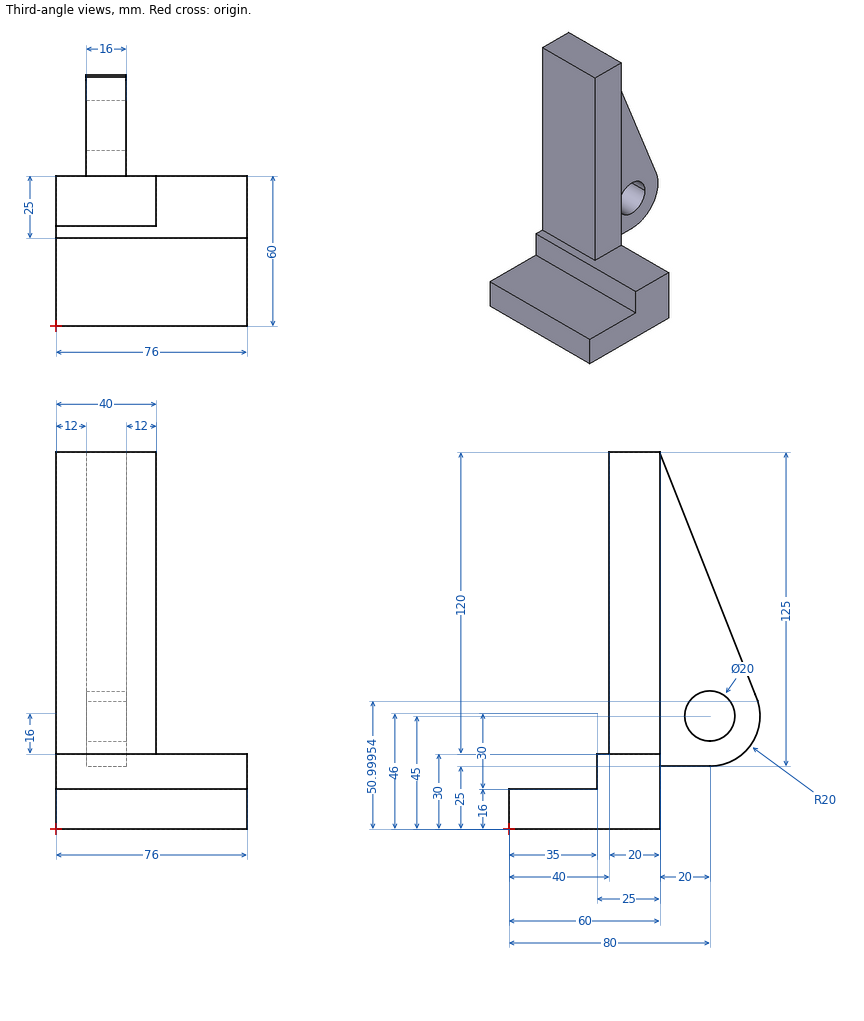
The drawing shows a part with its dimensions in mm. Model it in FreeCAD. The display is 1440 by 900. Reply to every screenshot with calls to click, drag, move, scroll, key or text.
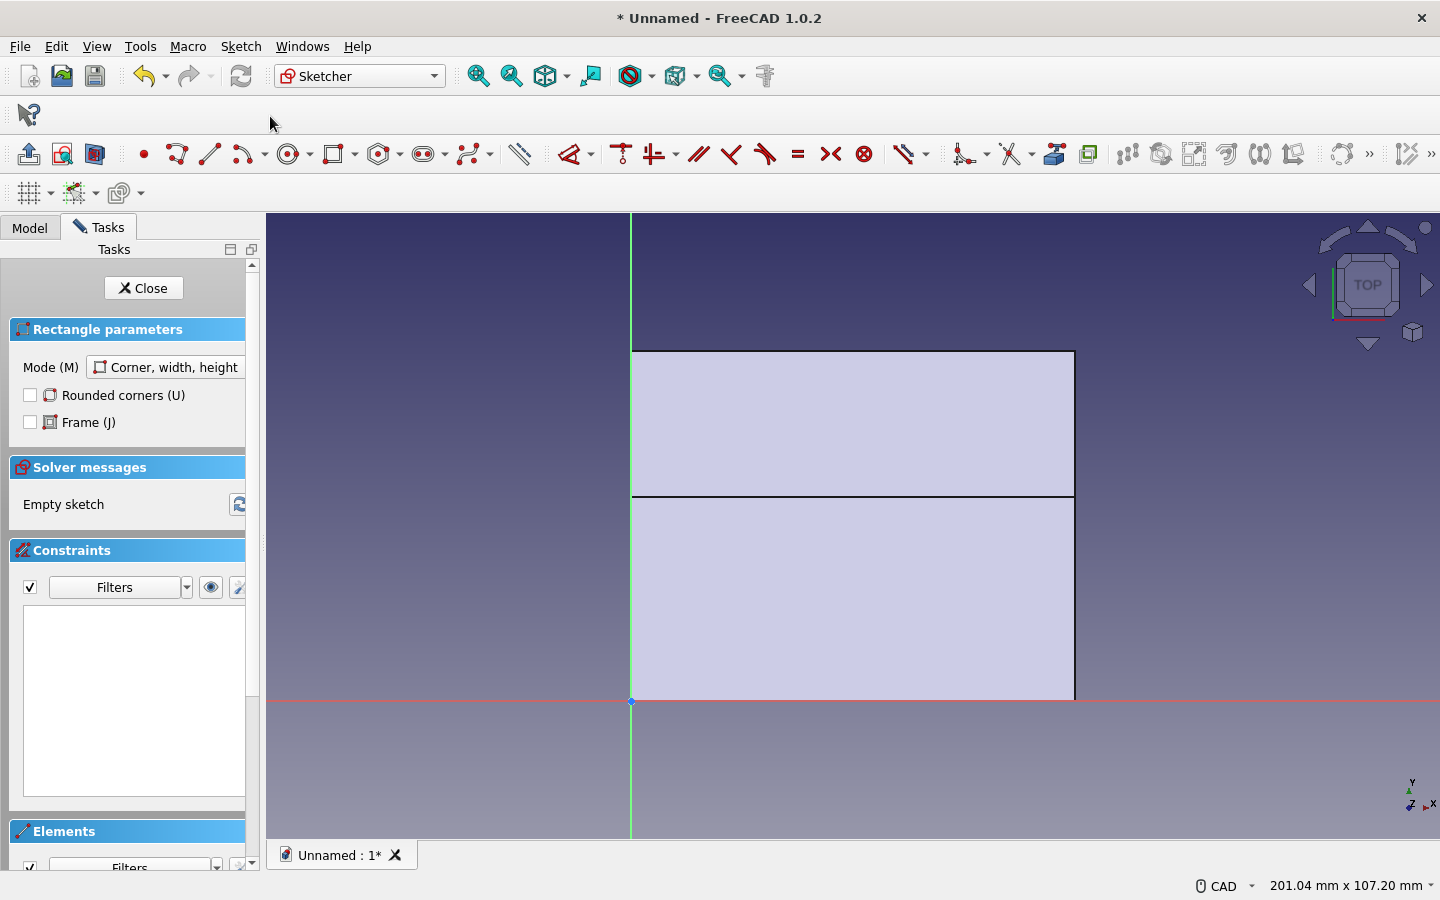
click(631, 351)
click(1075, 497)
key(Escape)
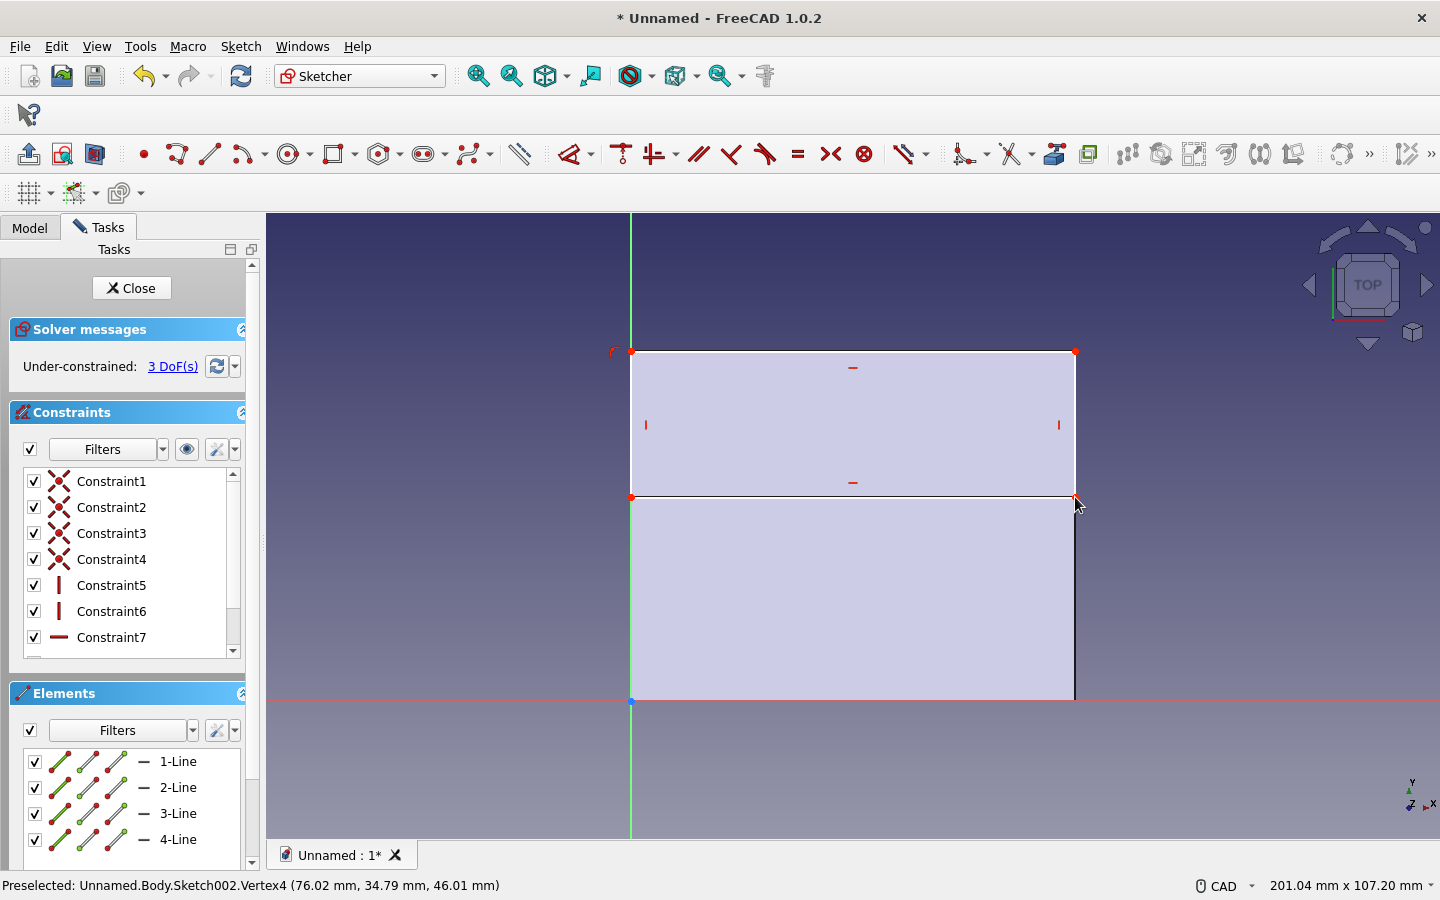
key(d)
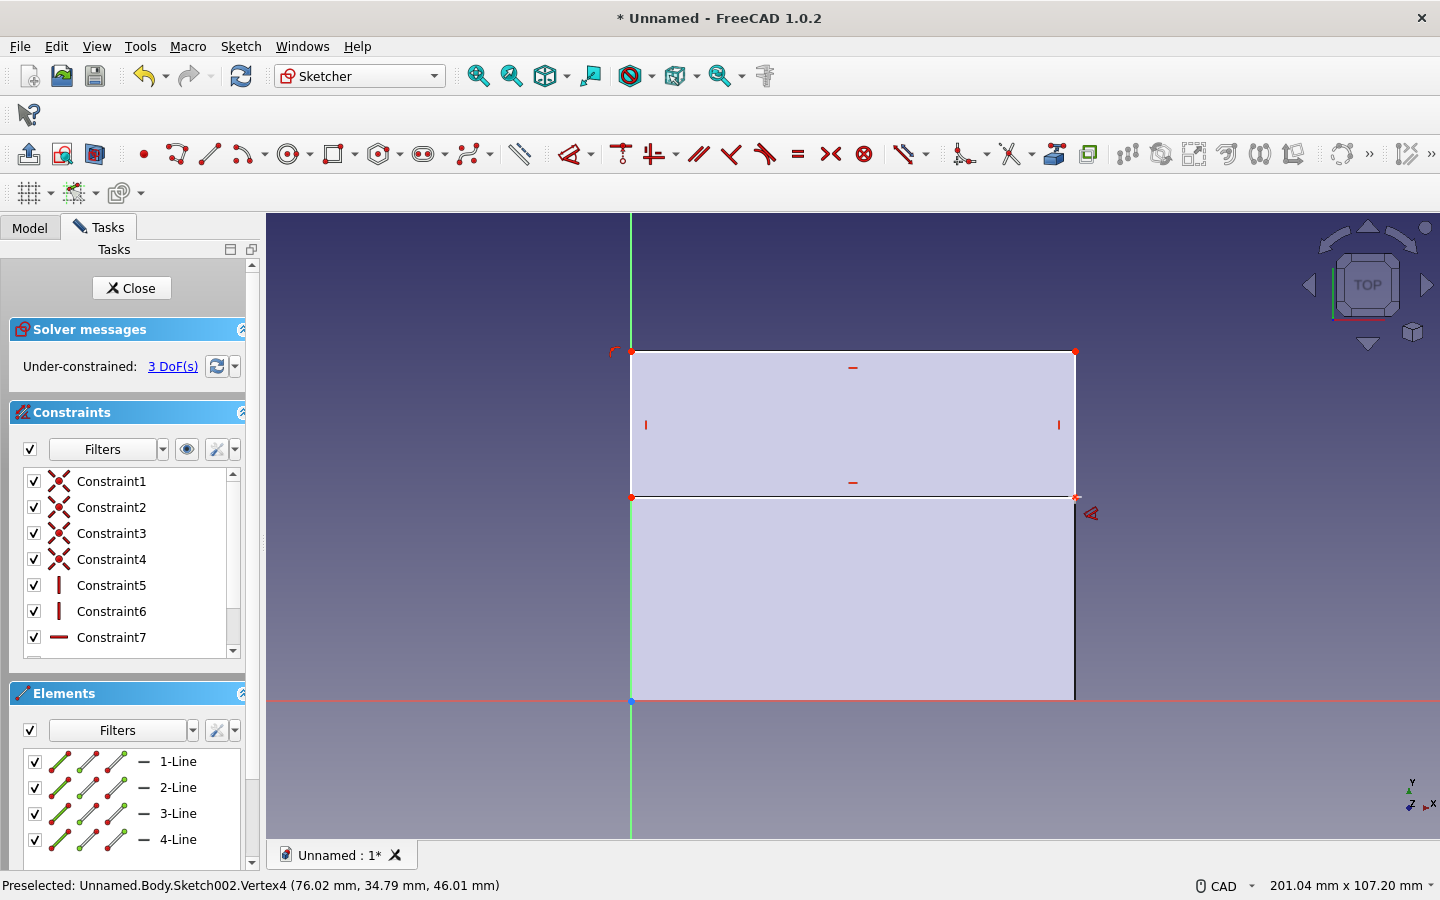
click(631, 396)
click(597, 425)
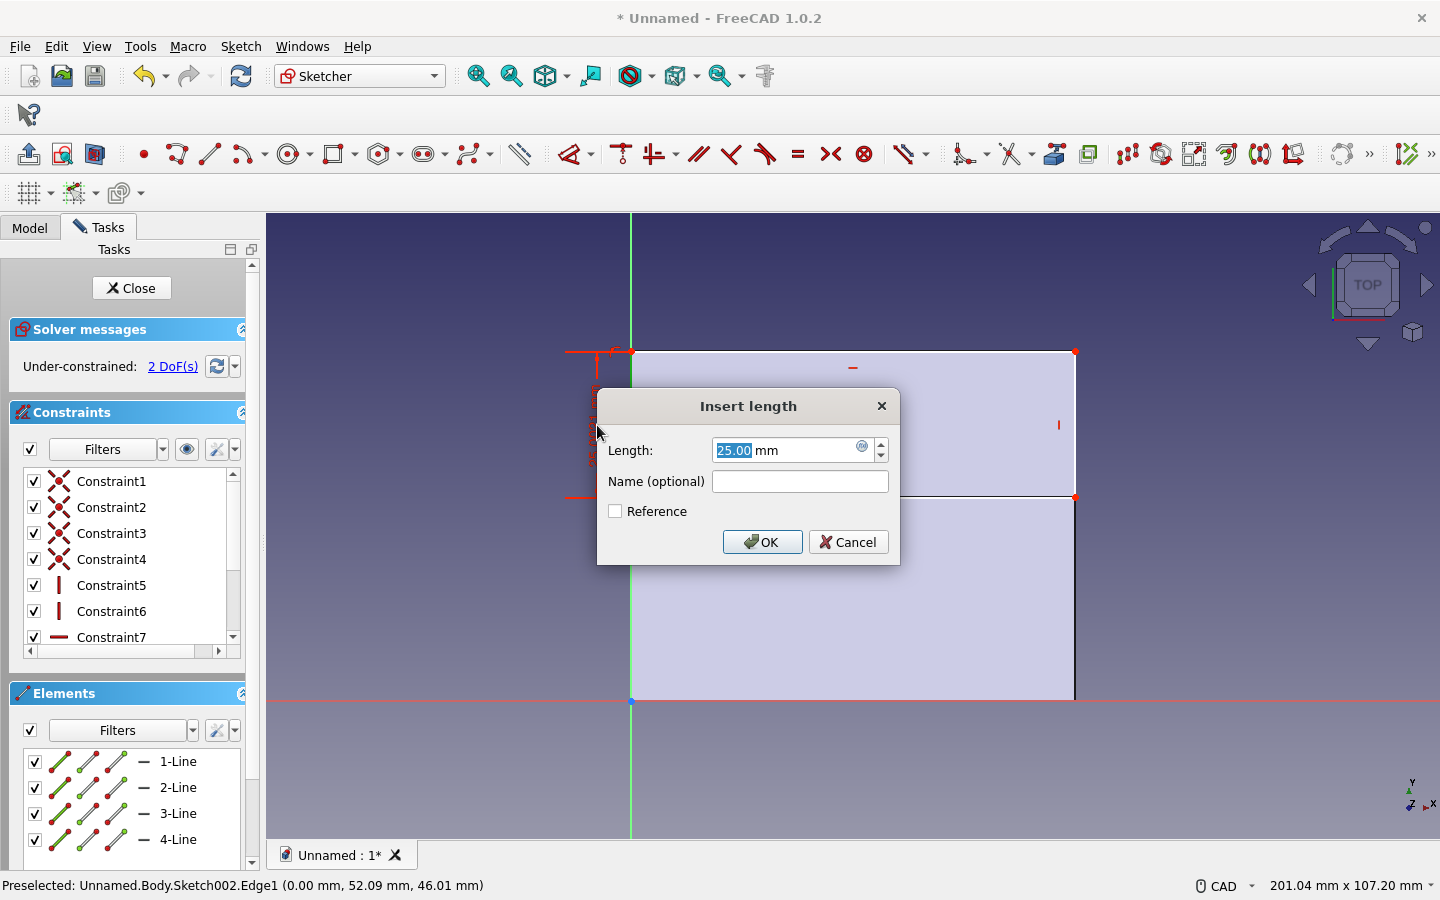
text(25)
key(Return)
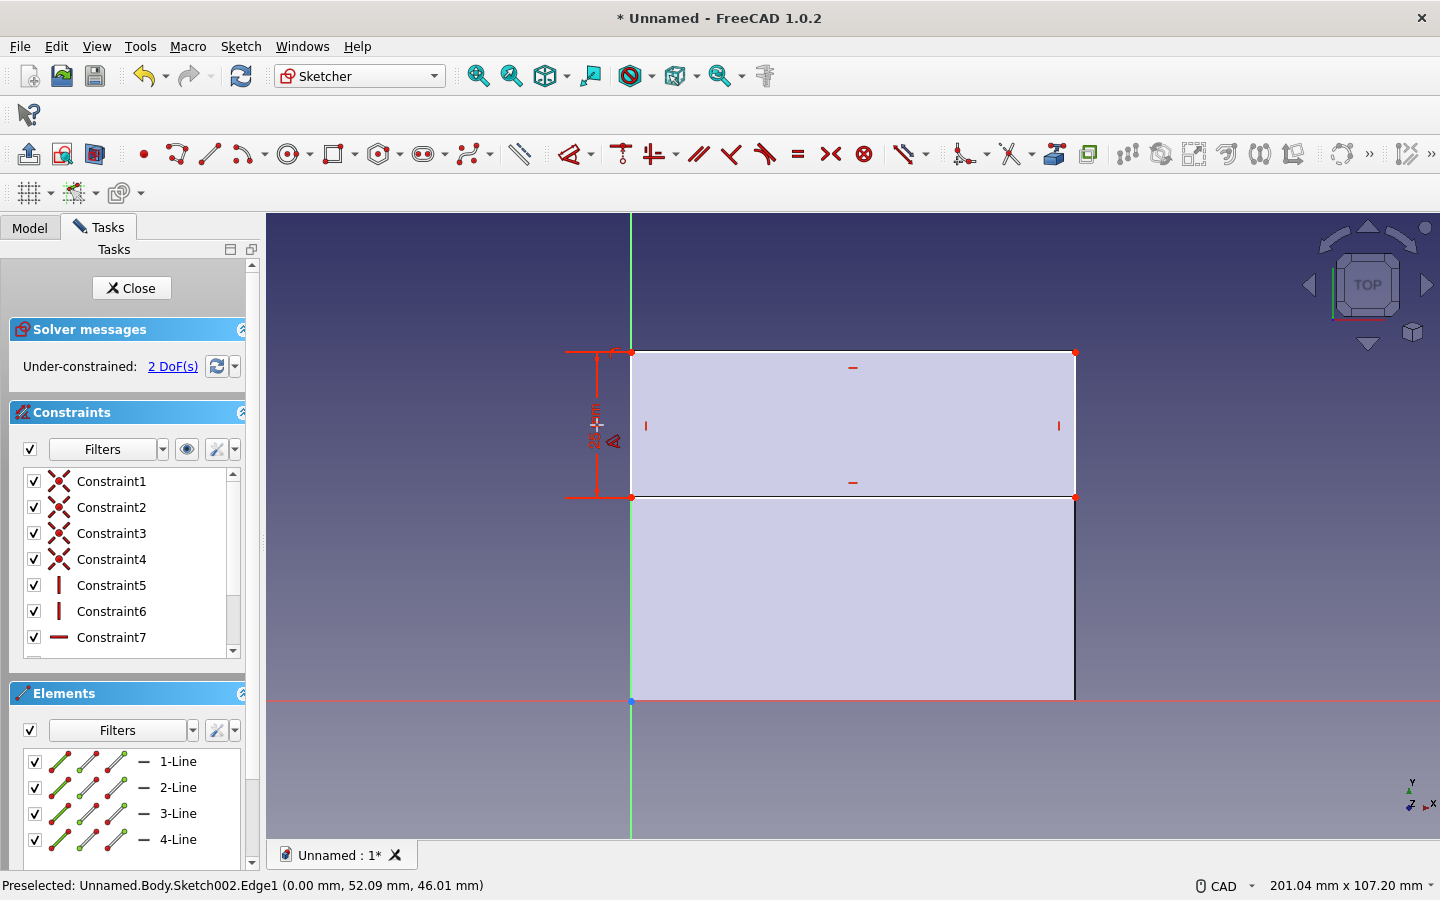
click(764, 498)
click(853, 464)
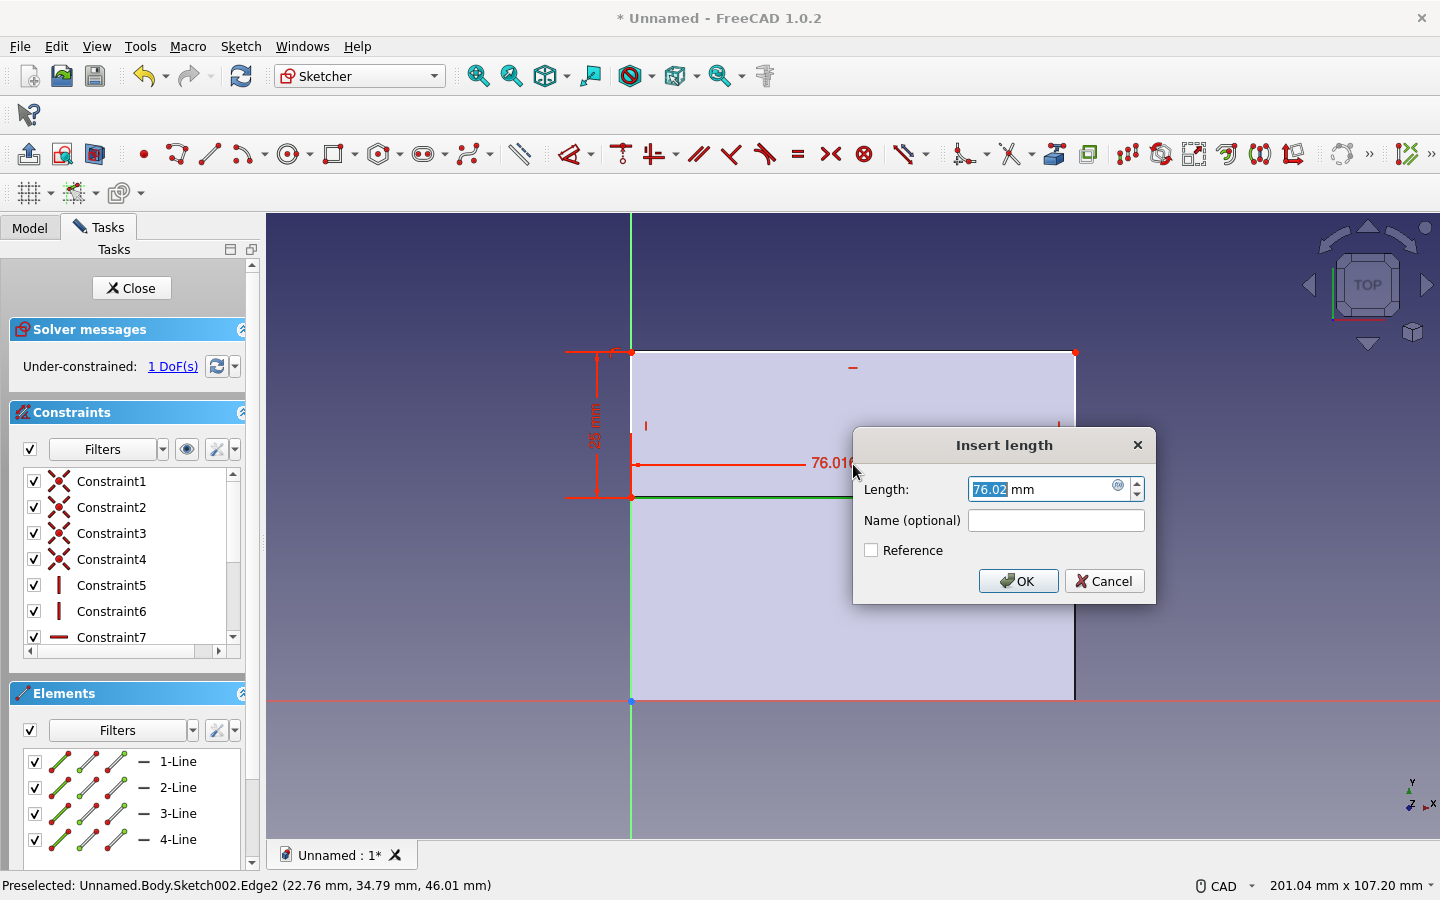
text(76)
key(Return)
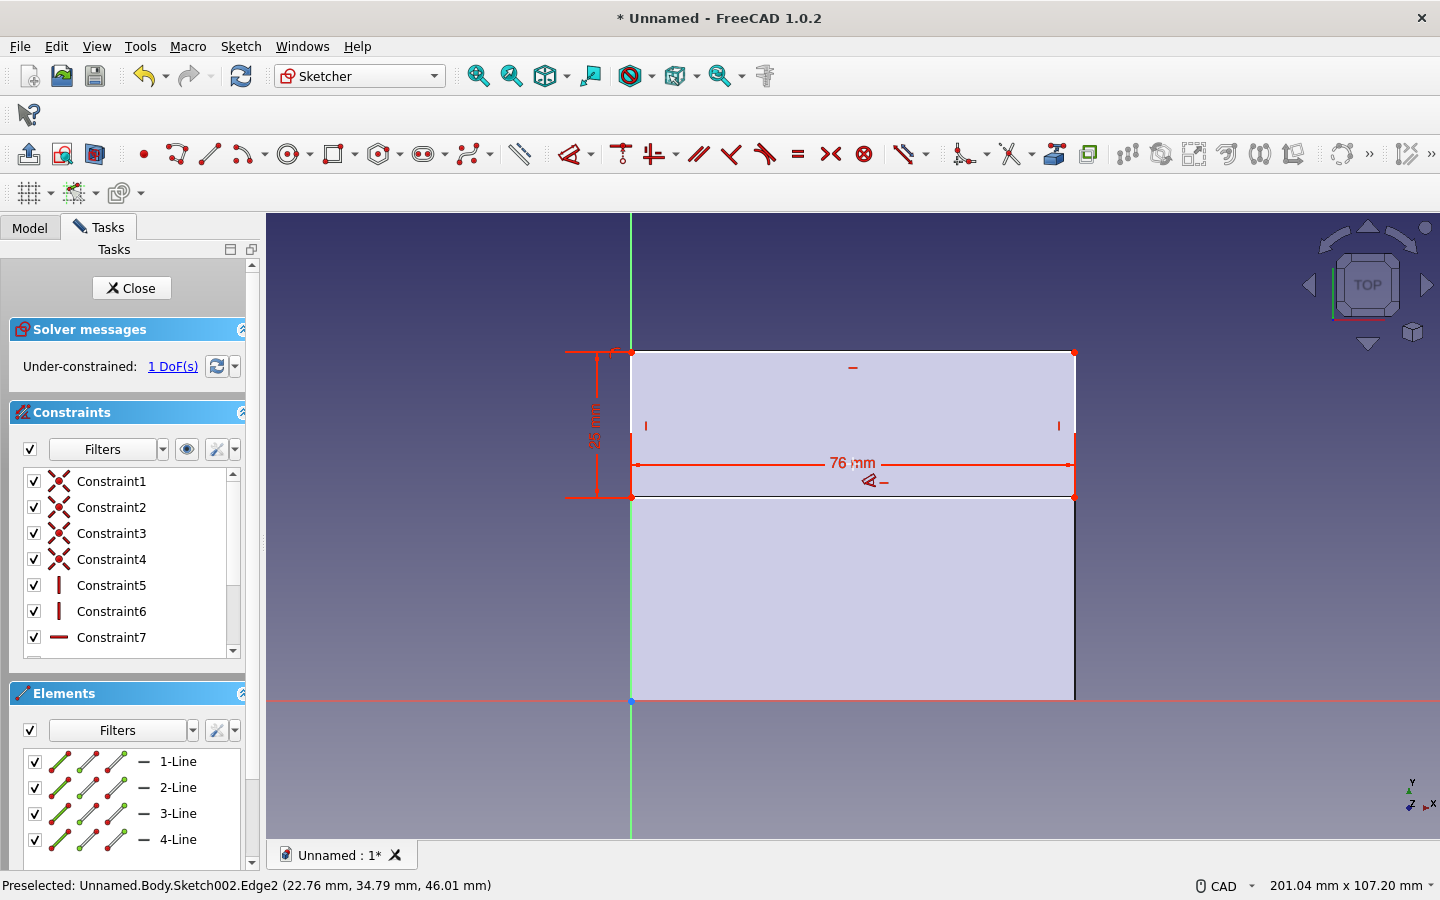
click(631, 352)
click(597, 527)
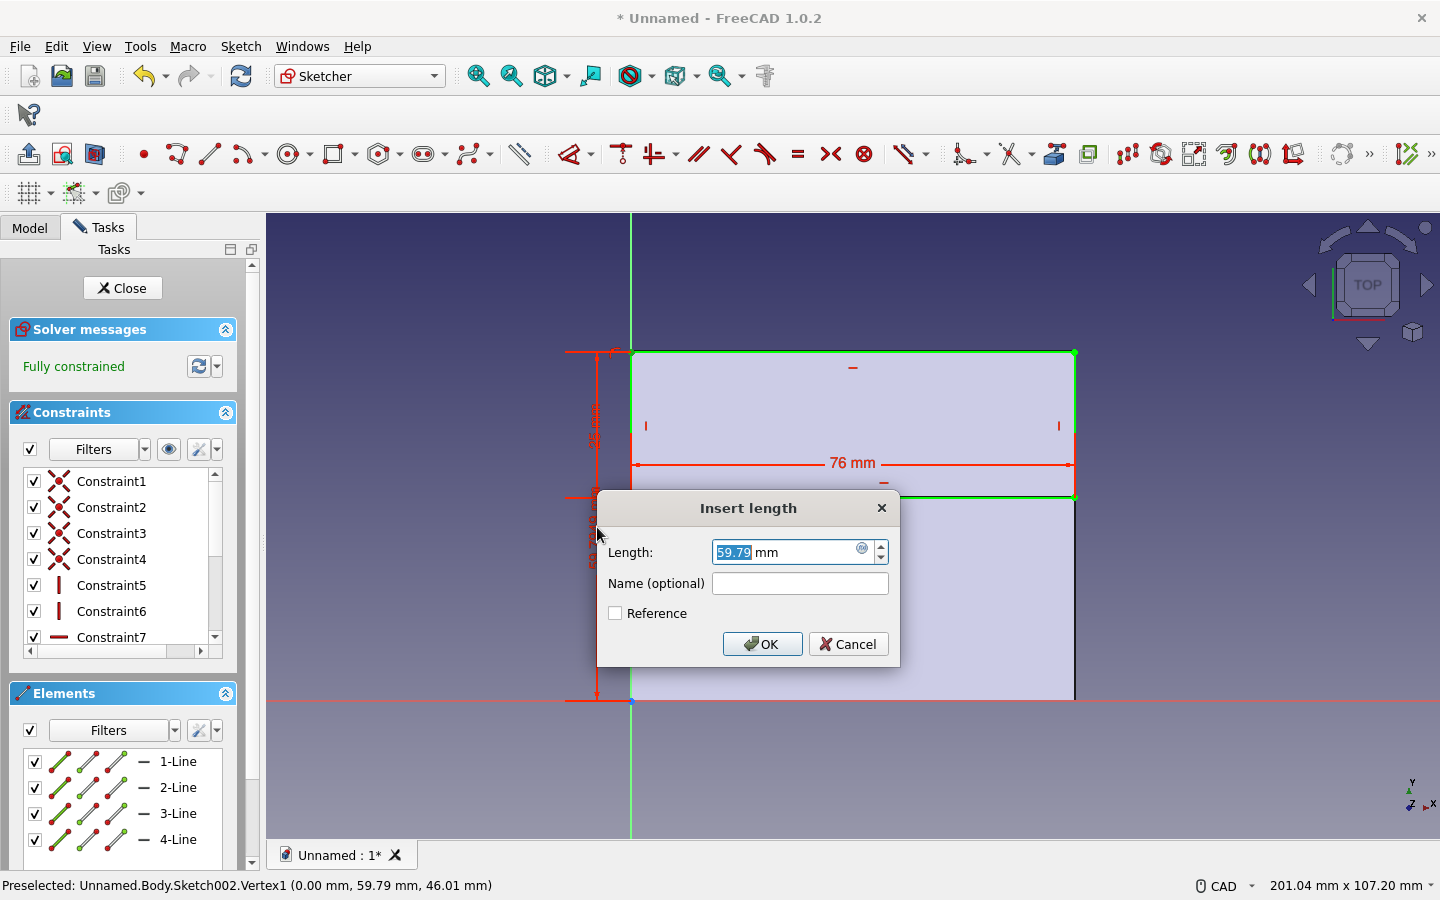
text(60)
key(Return)
key(Escape)